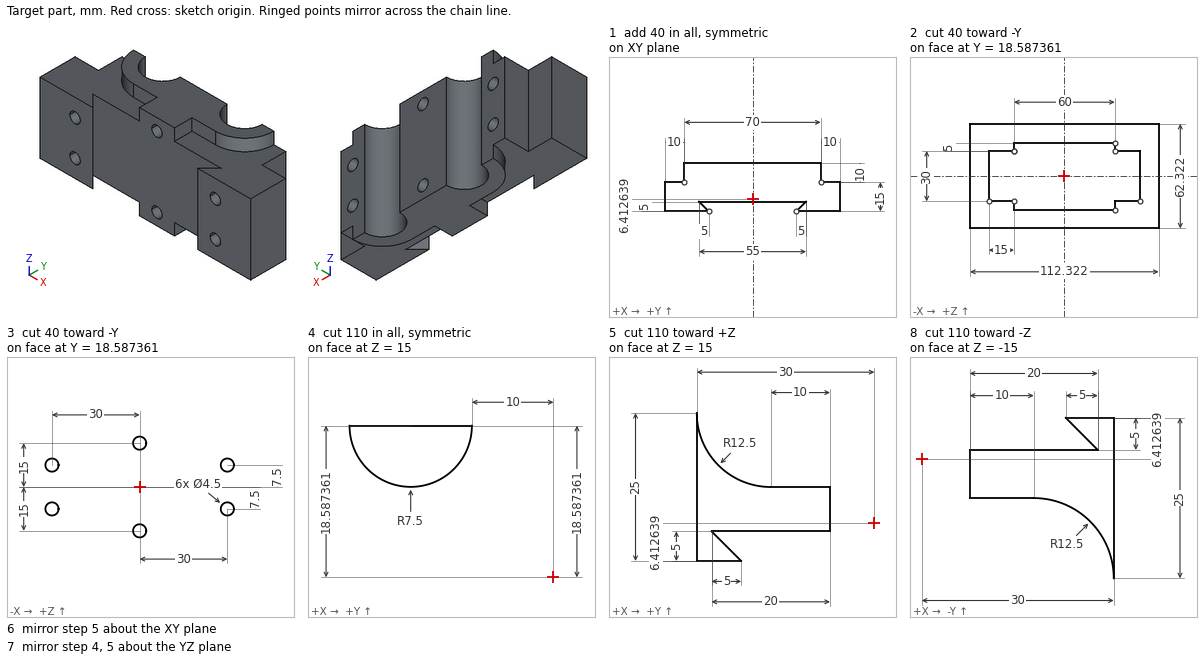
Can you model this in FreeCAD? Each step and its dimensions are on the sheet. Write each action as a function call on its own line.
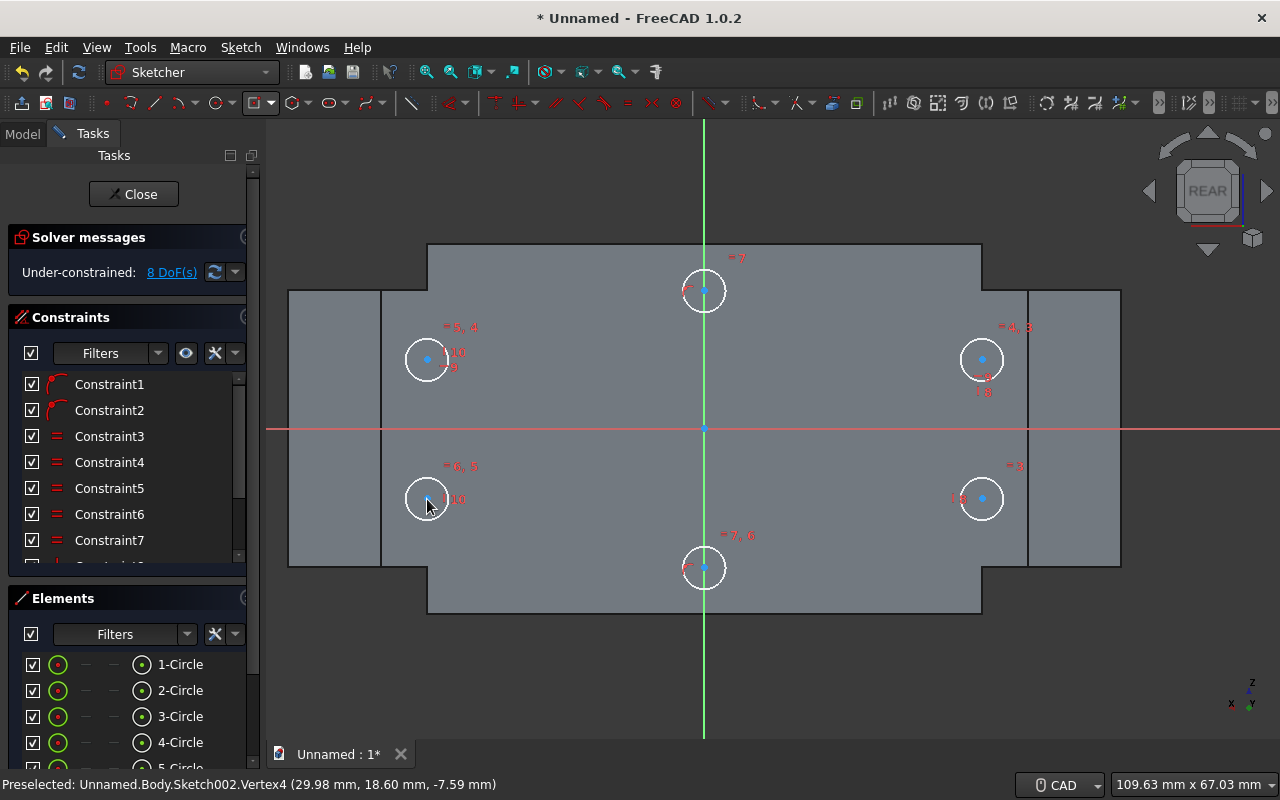
click(982, 499)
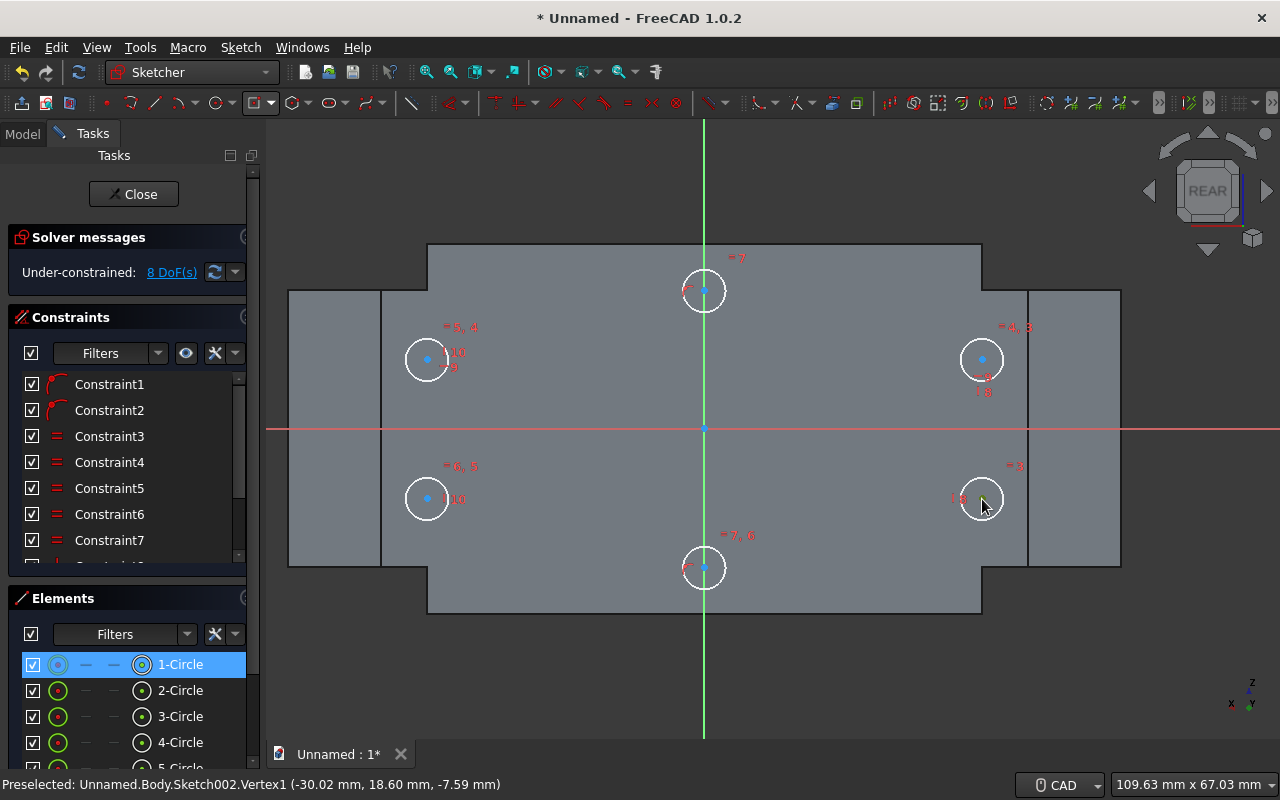
click(427, 499)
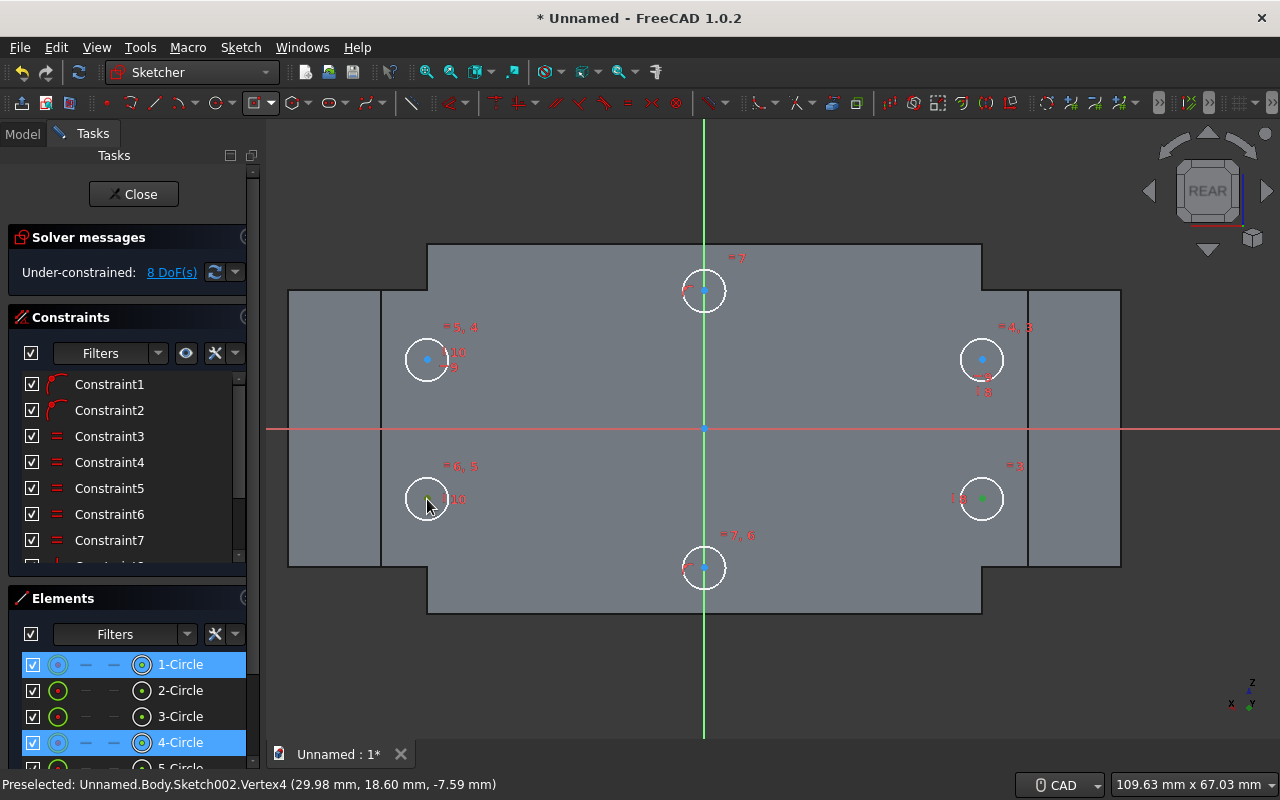
key(h)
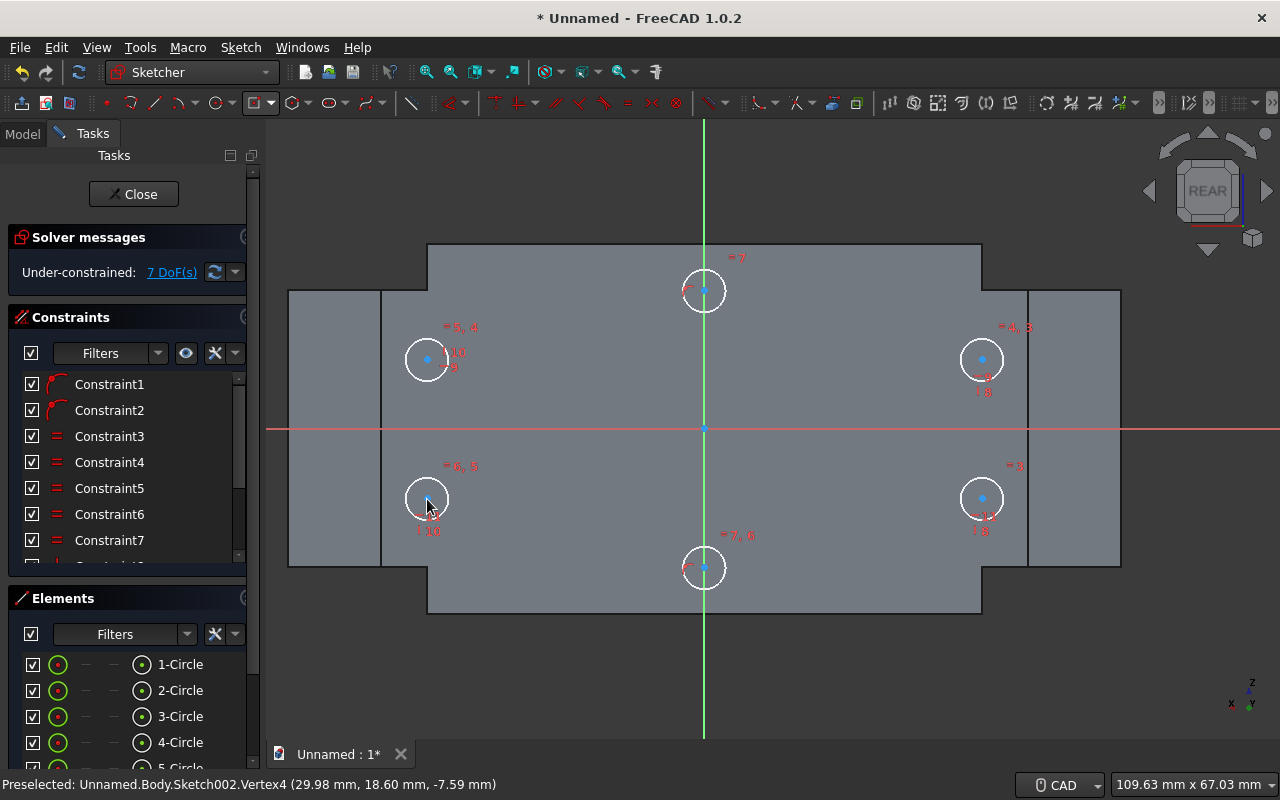
key(d)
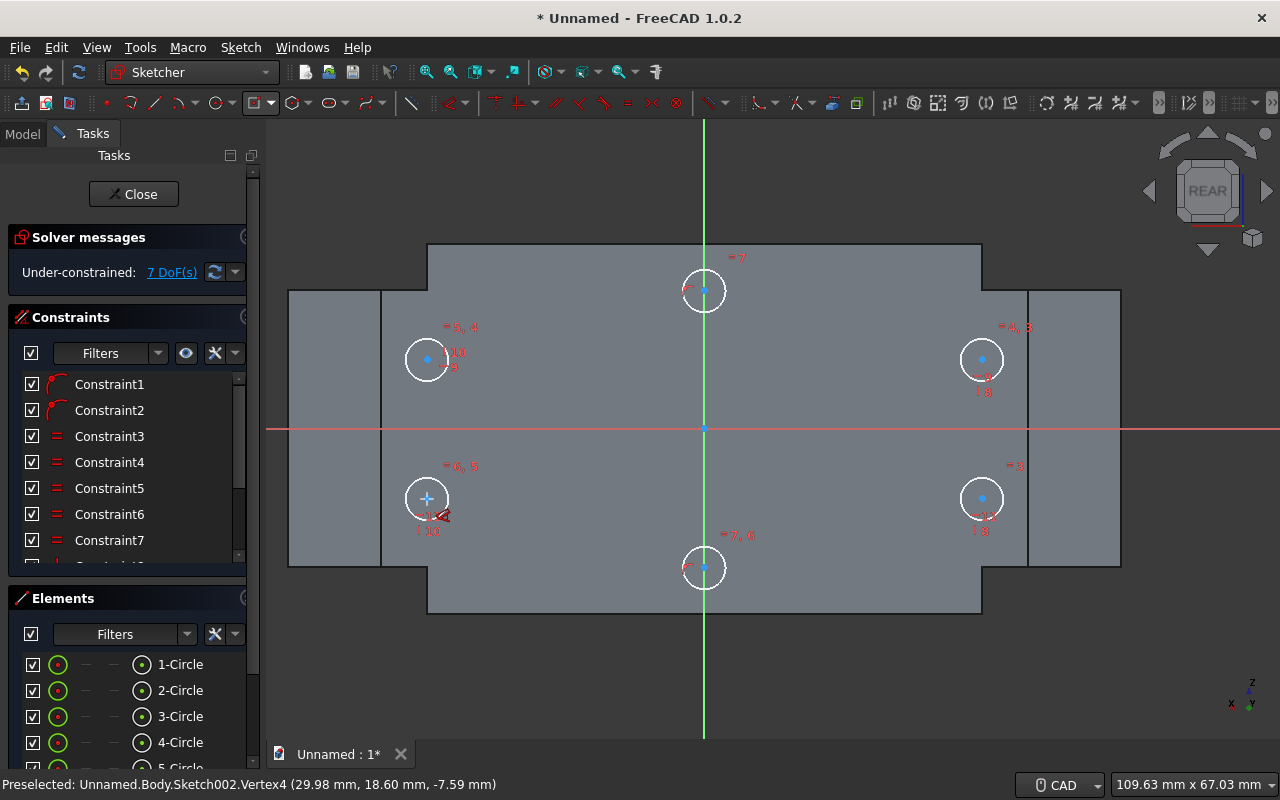
click(997, 484)
click(1020, 461)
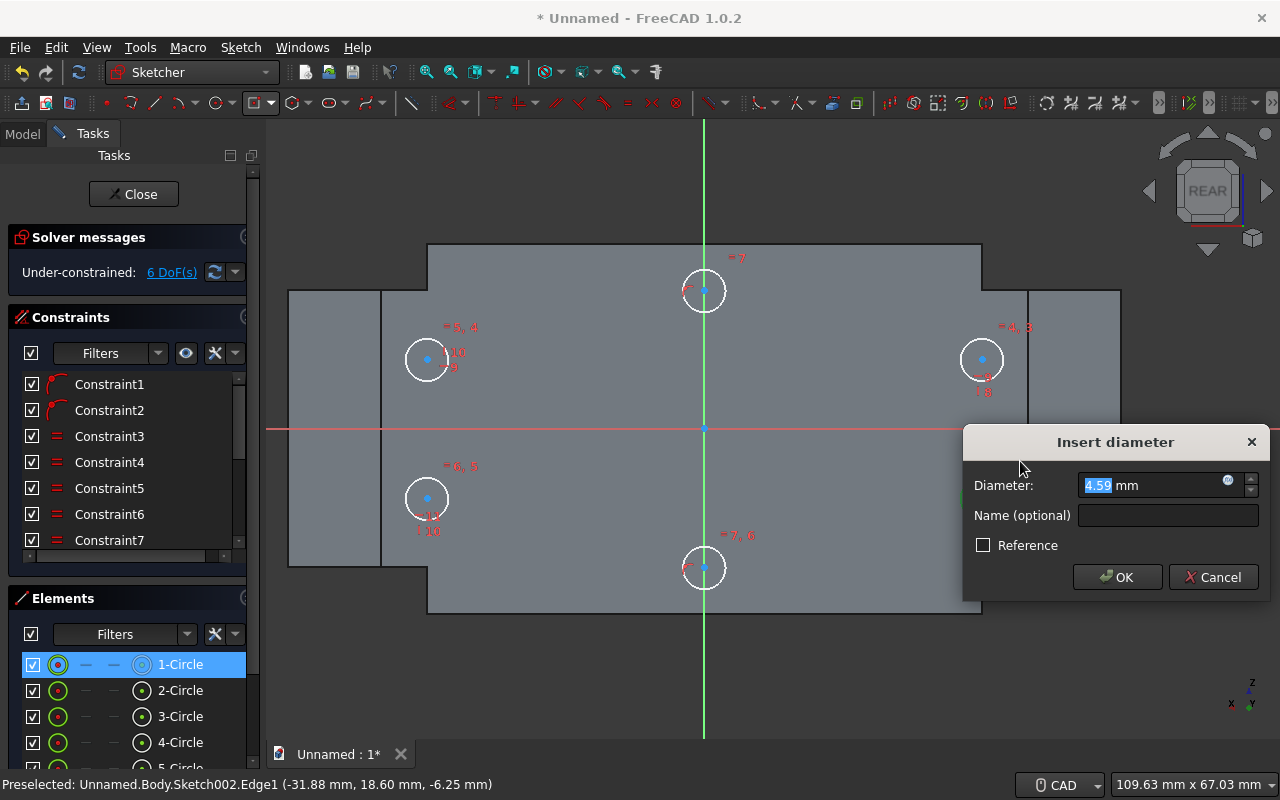
text(4.5)
key(Return)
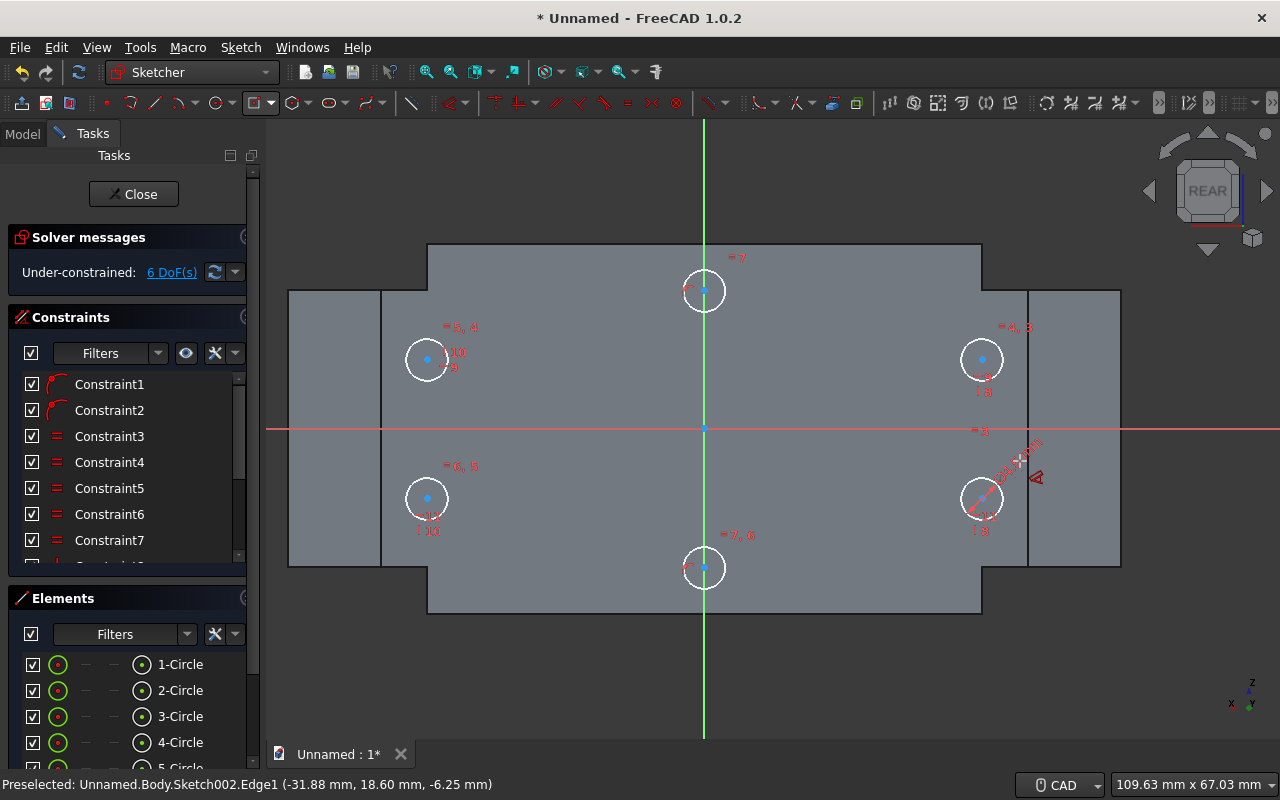
click(982, 499)
click(843, 533)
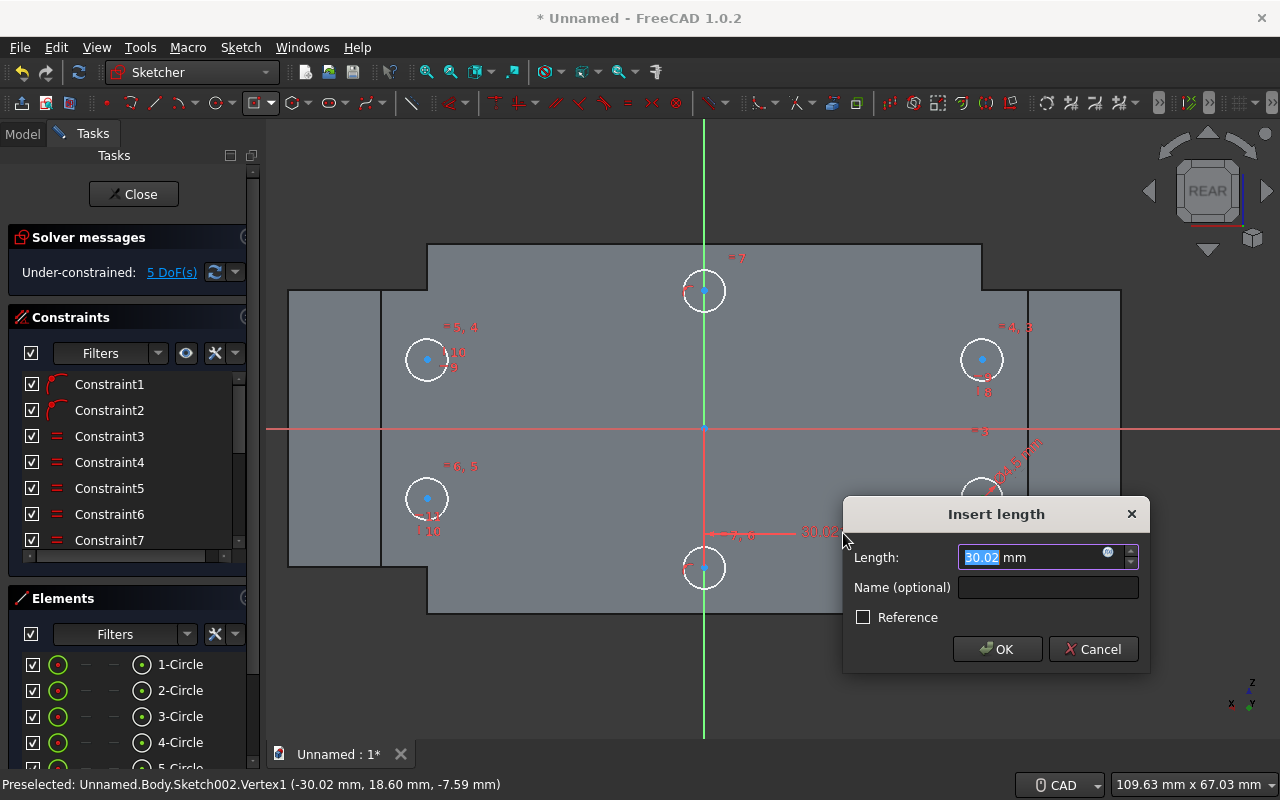
text(30)
key(Return)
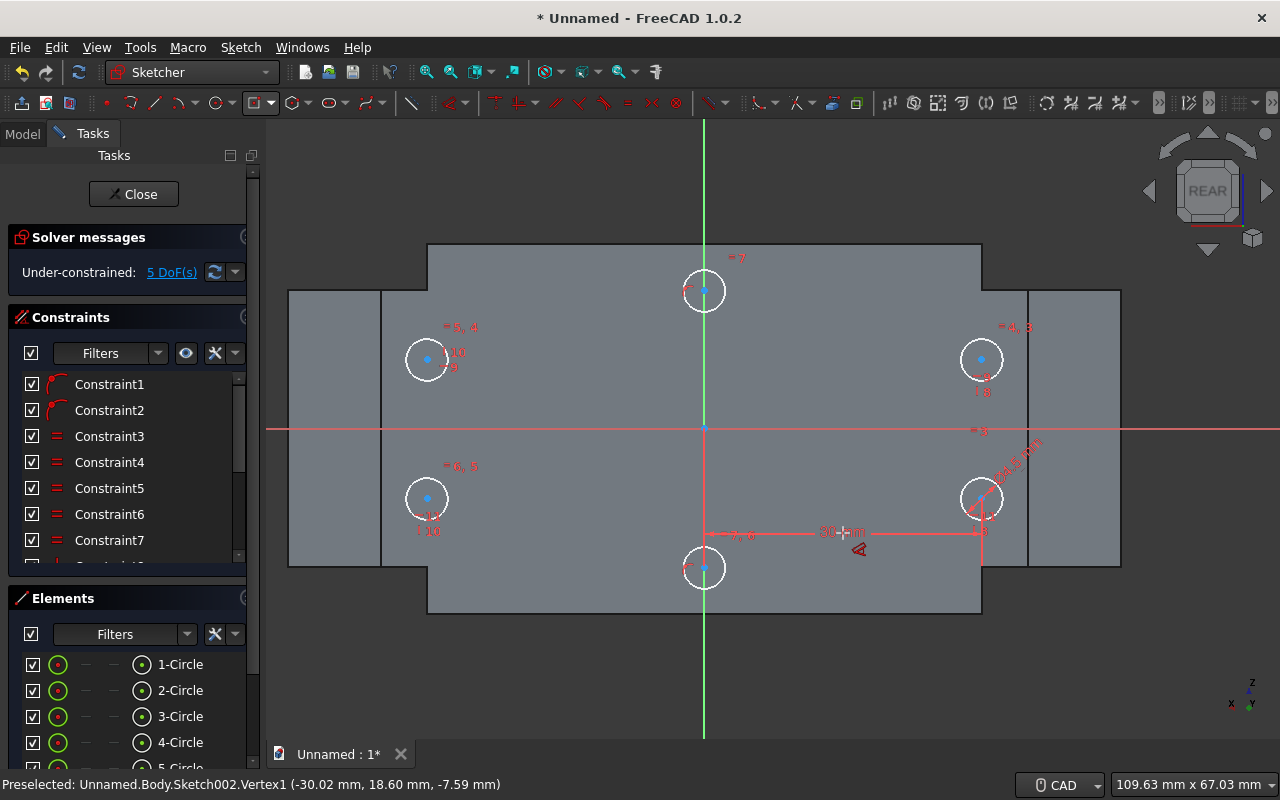
click(427, 360)
click(566, 326)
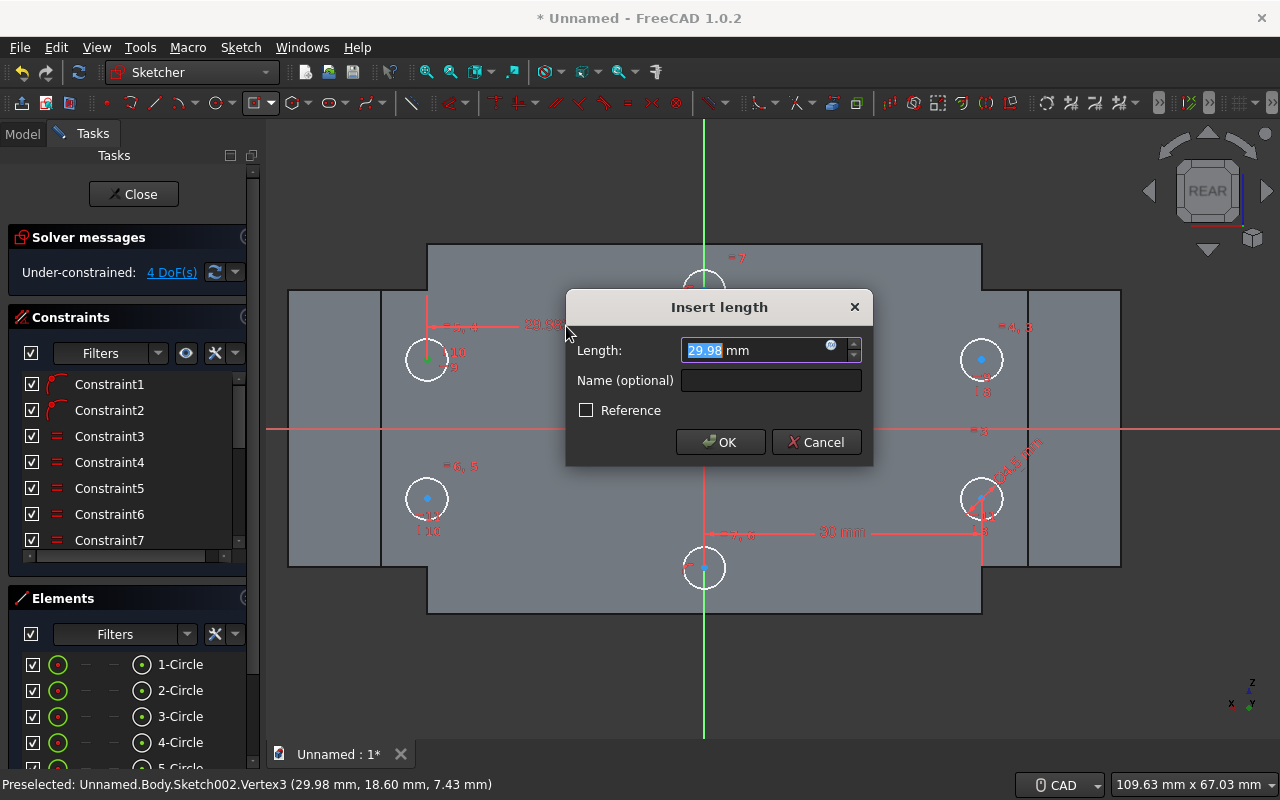
text(30)
key(Return)